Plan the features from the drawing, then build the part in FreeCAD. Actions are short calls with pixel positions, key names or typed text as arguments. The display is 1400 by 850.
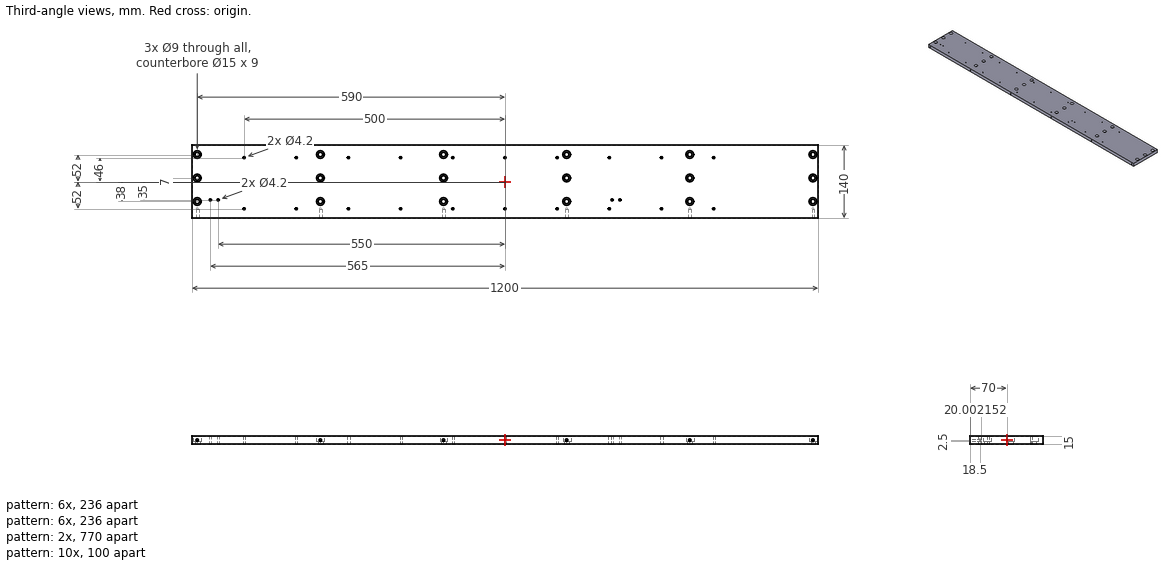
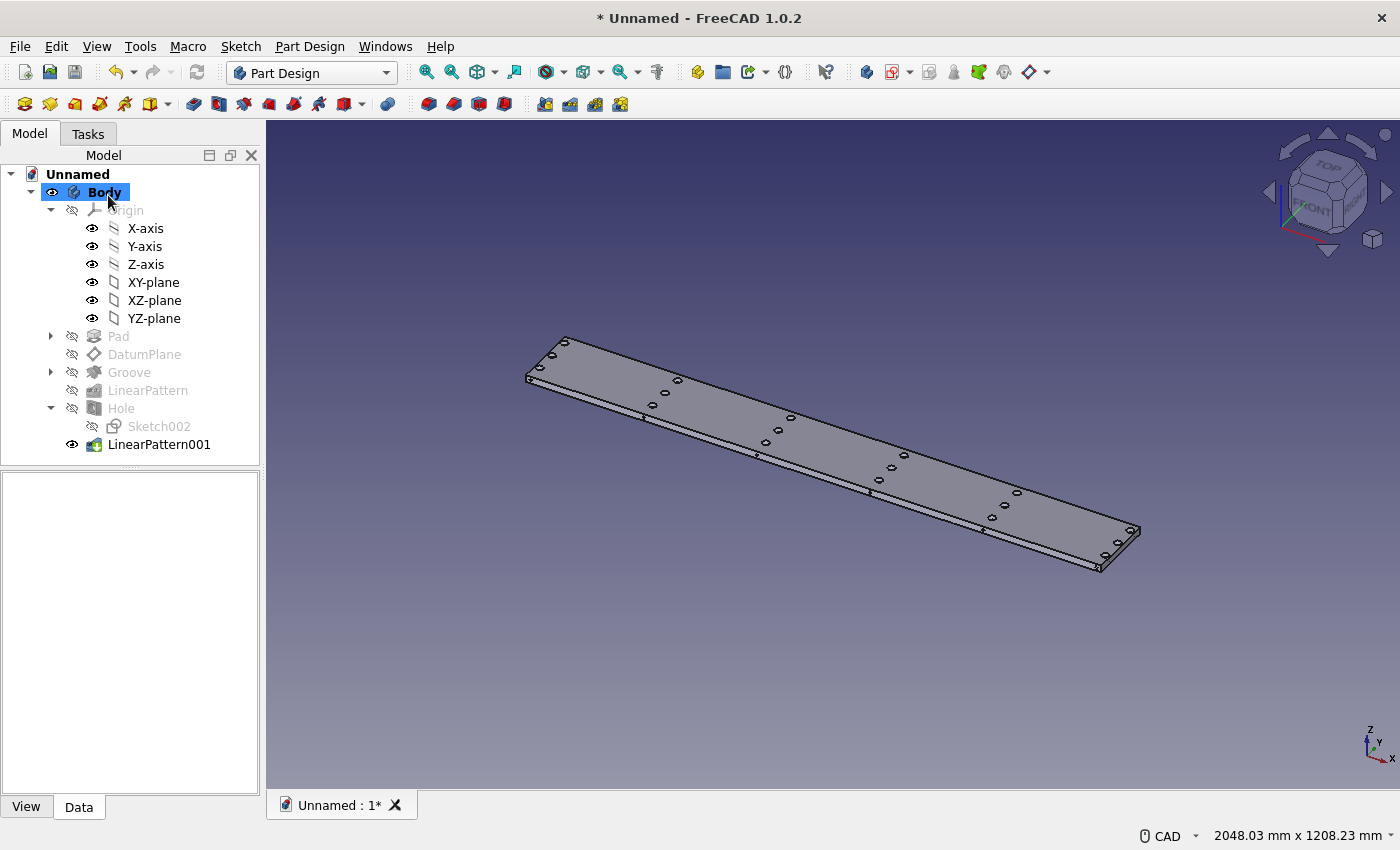
key(5)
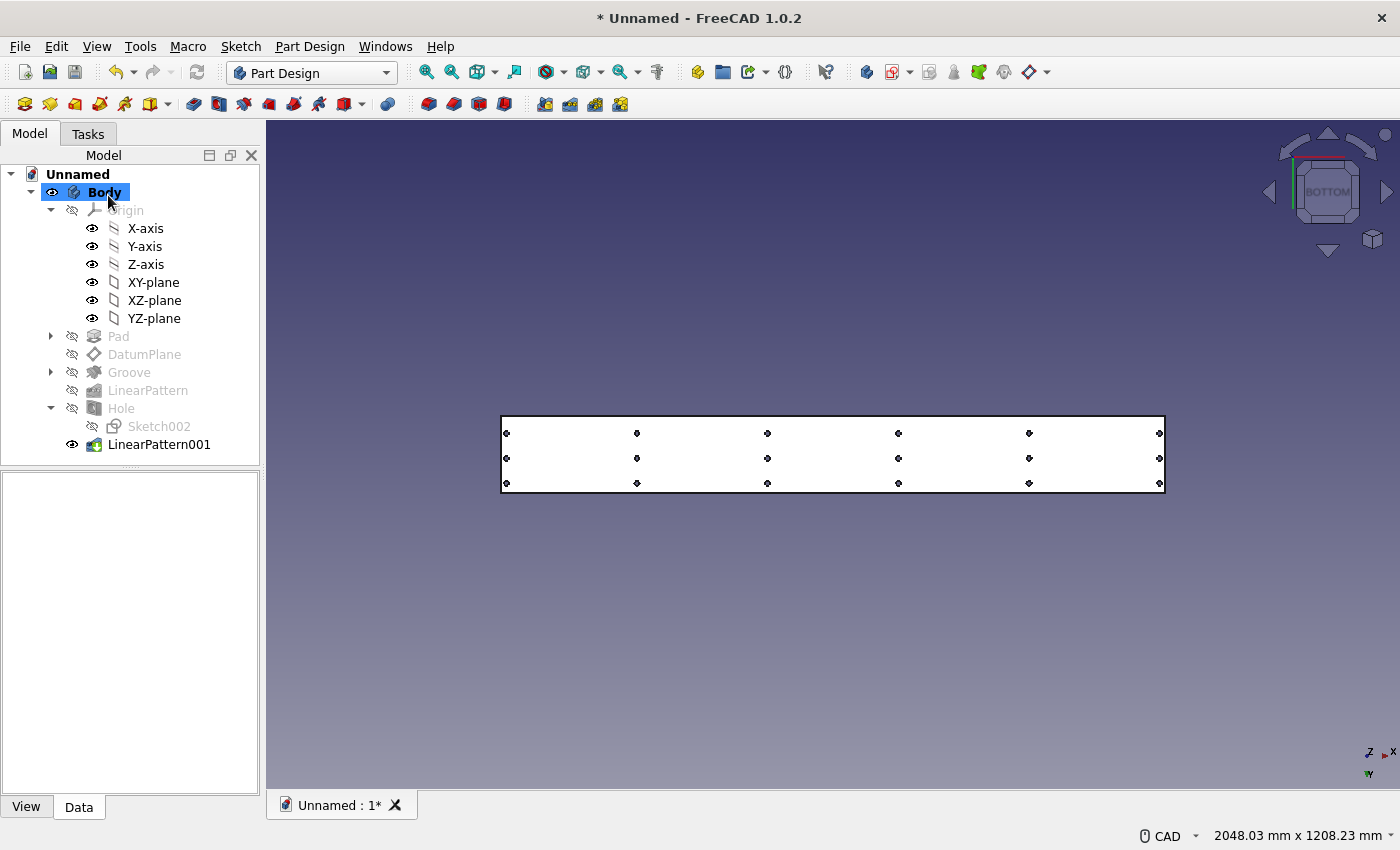
click(1118, 453)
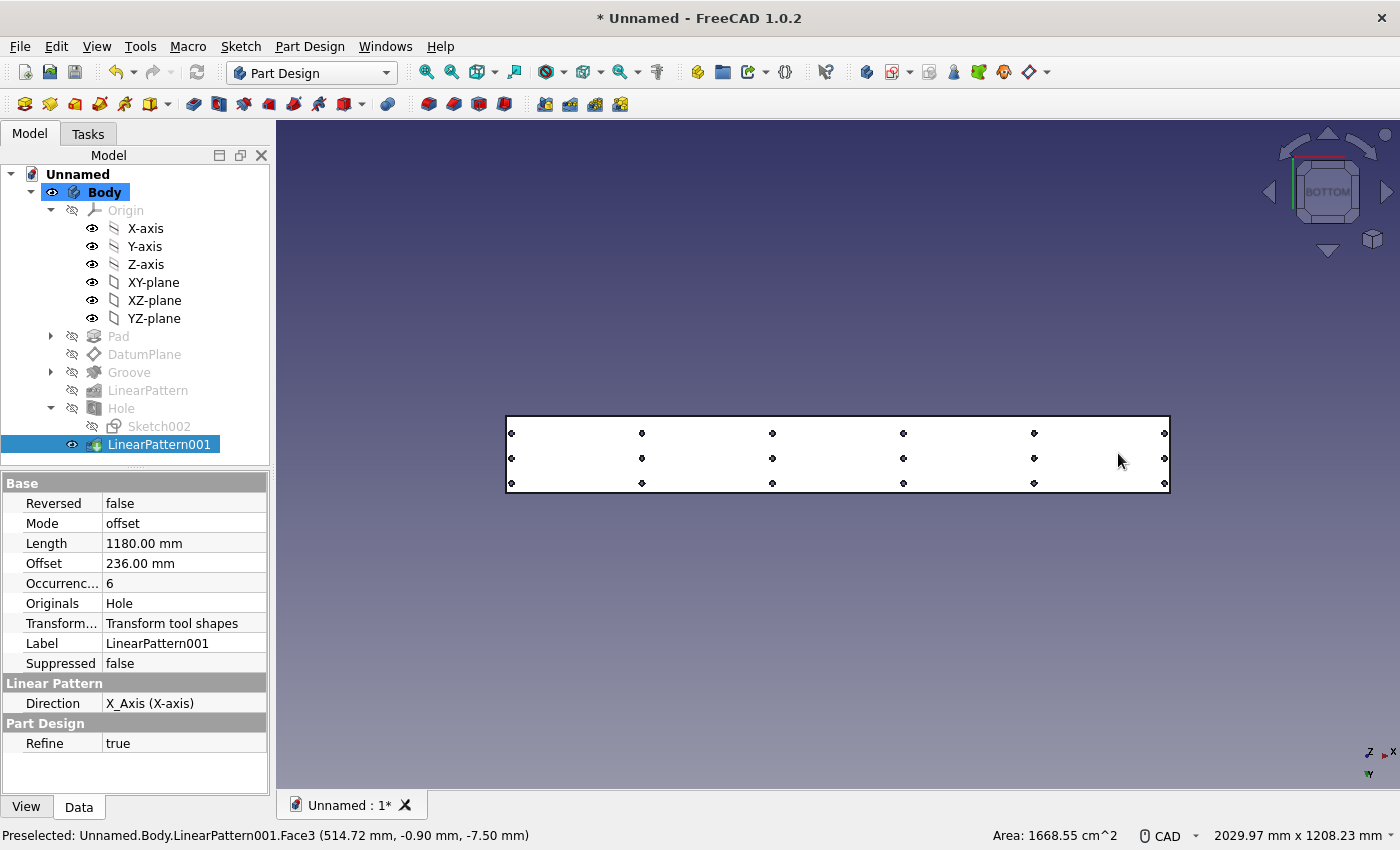
click(892, 72)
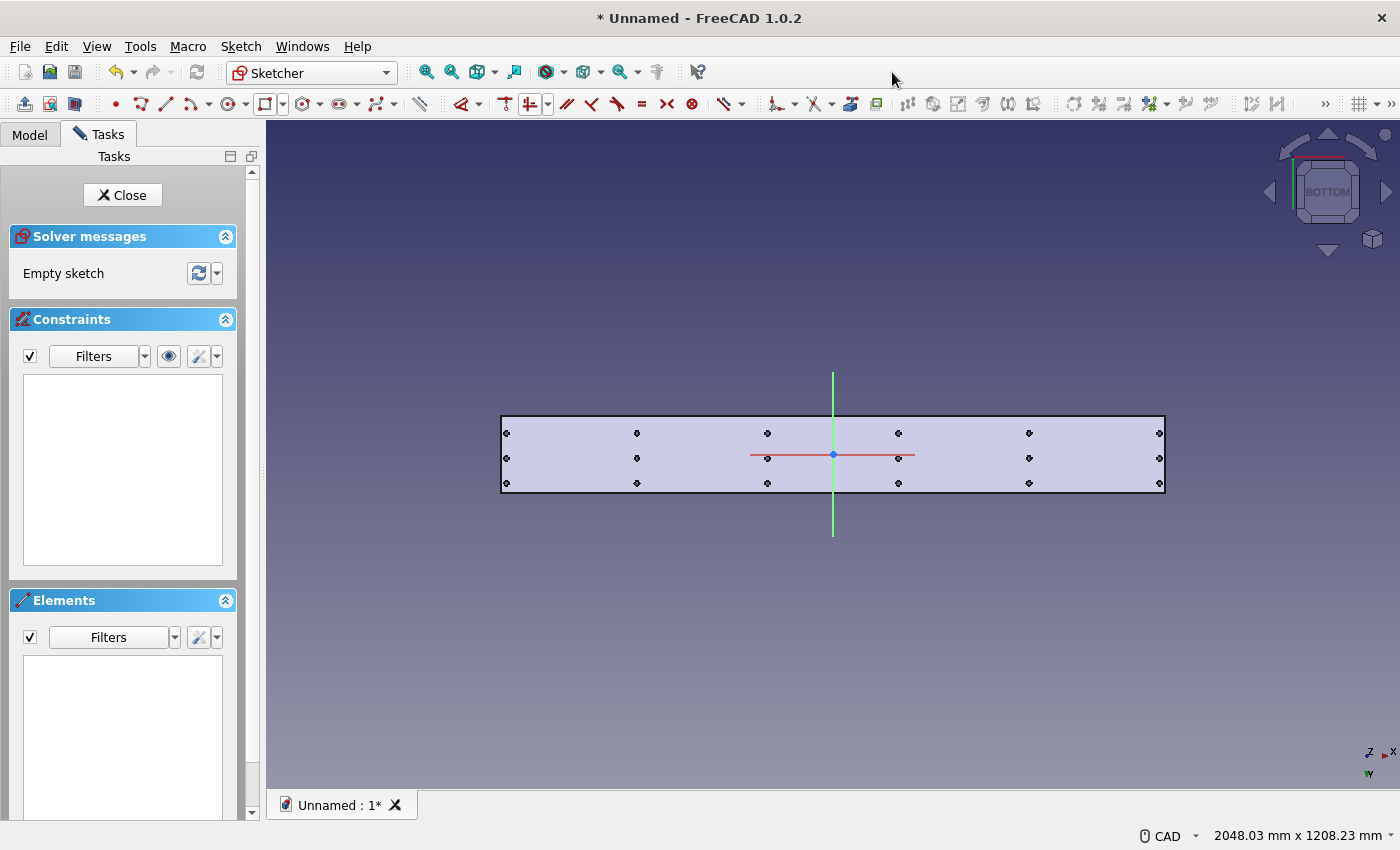
scroll(512, 434, up, 15)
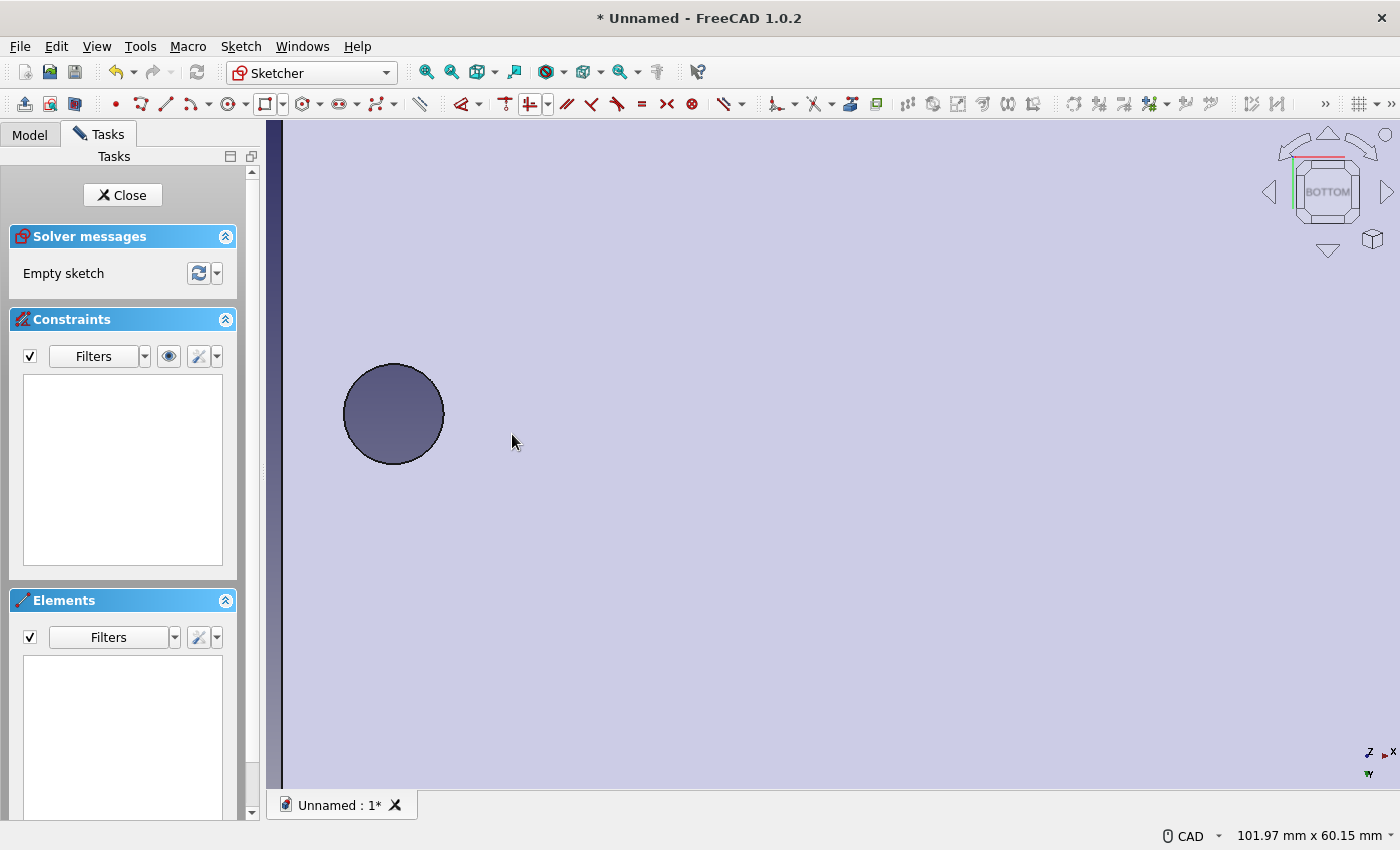
scroll(751, 445, up, 6)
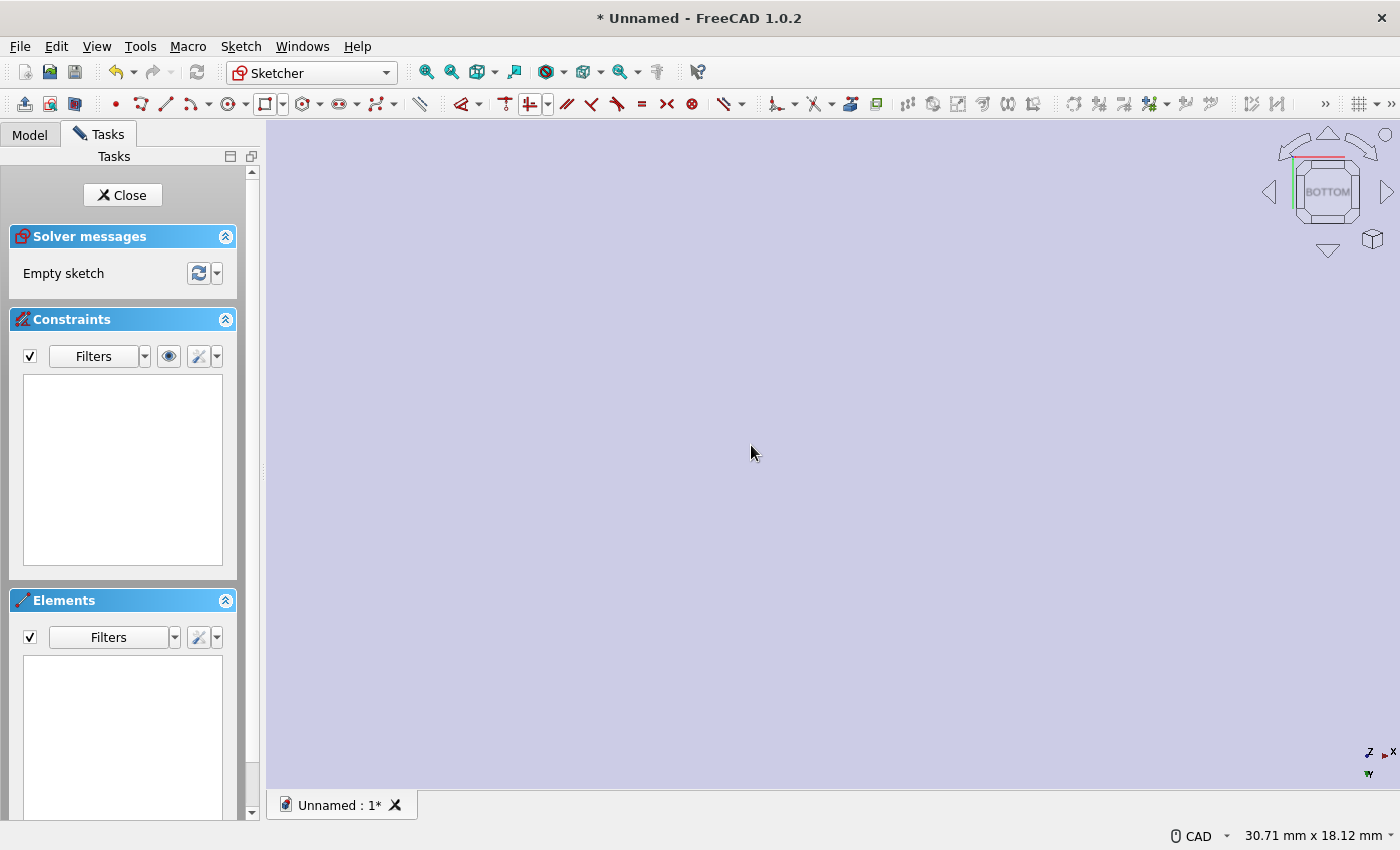
click(228, 104)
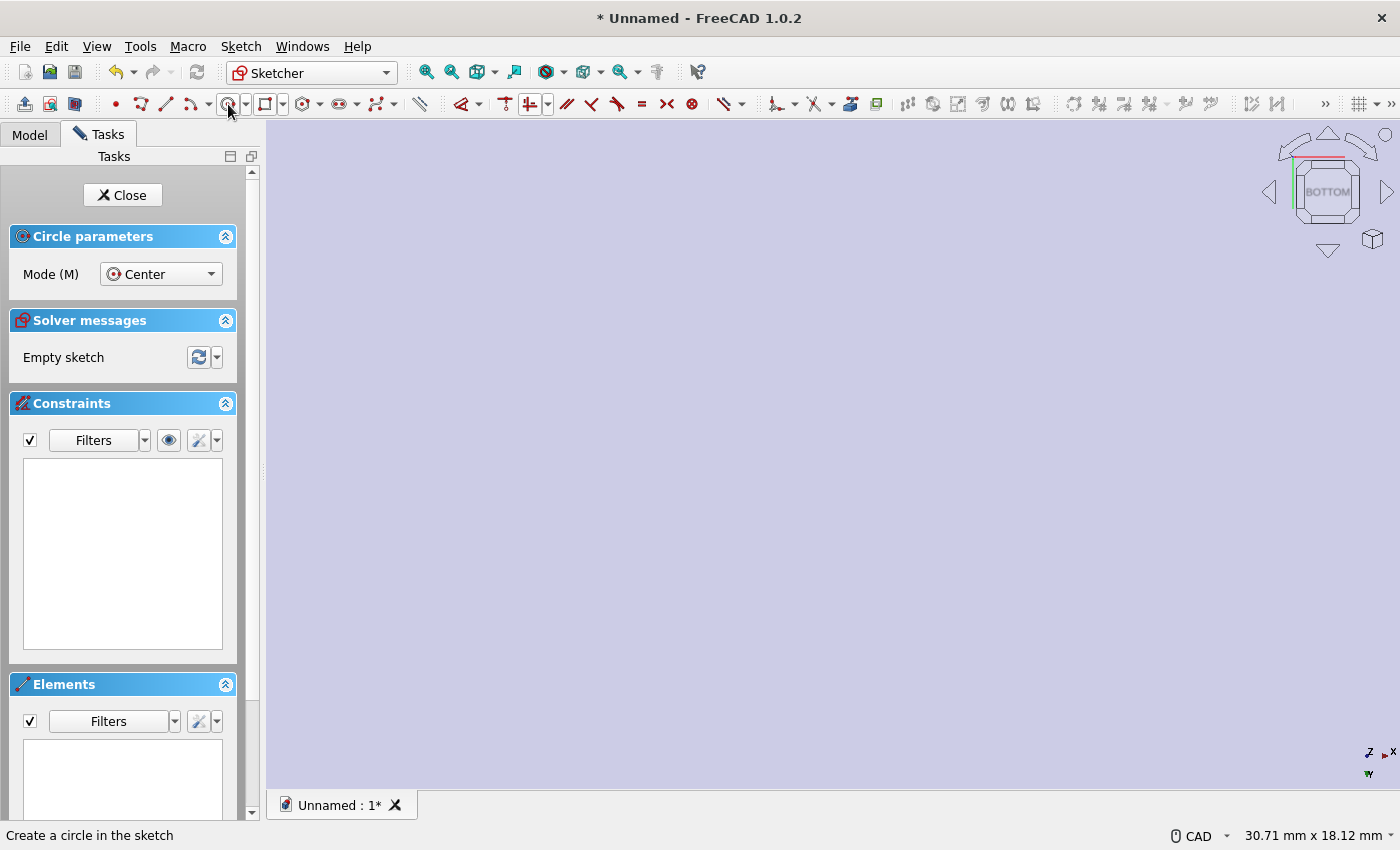
click(1041, 452)
move(1096, 397)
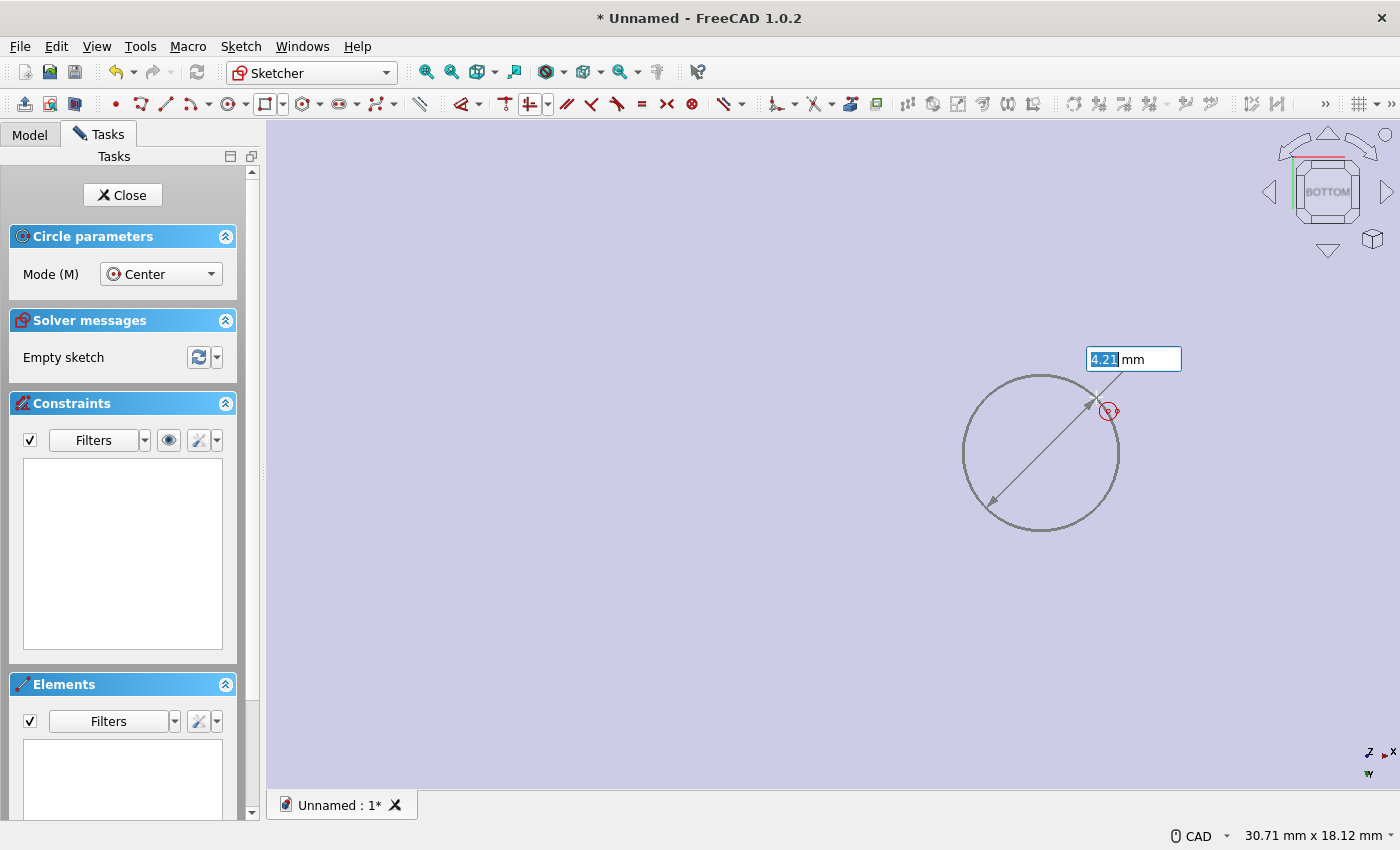
text(4.2)
key(Return)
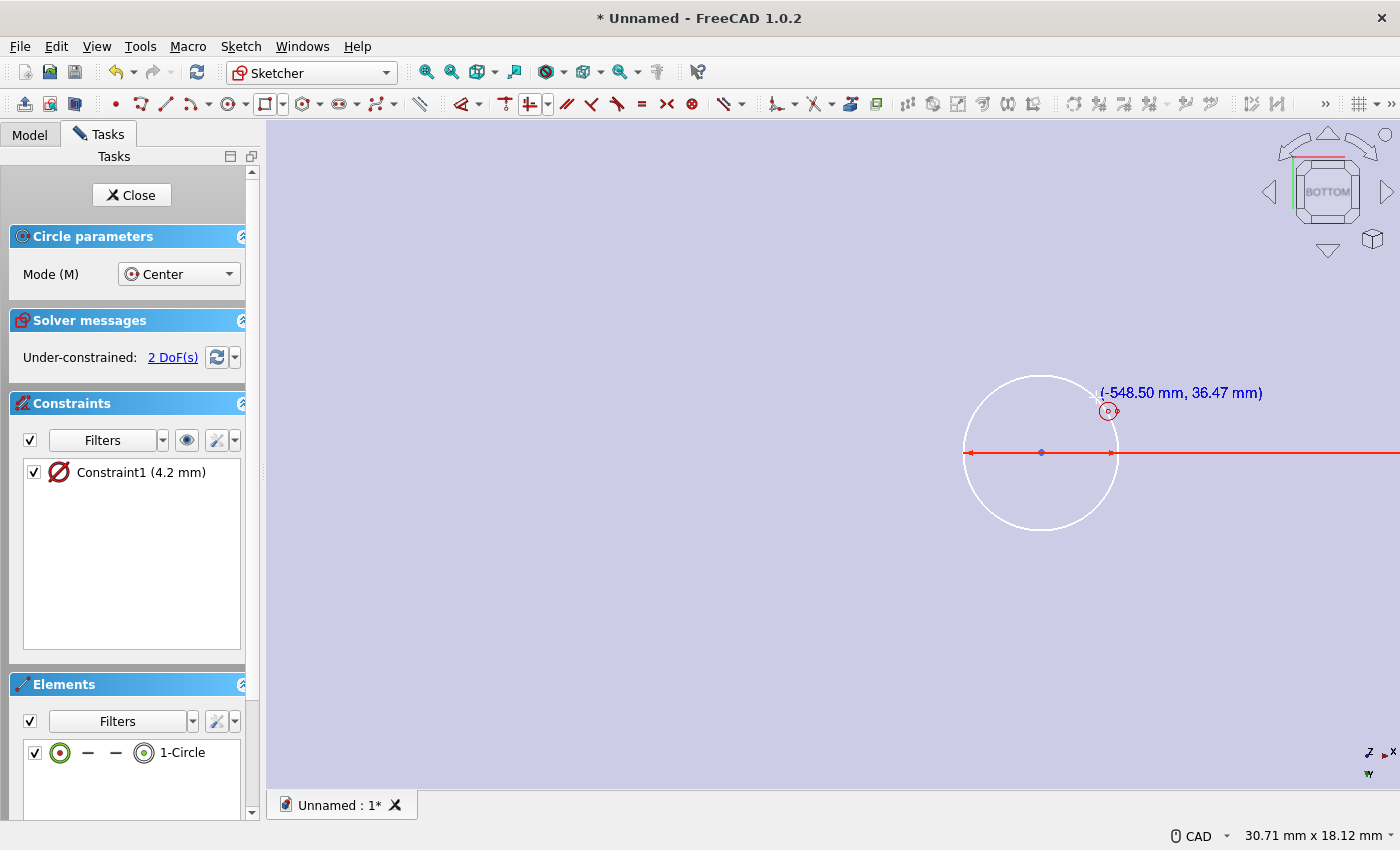
click(487, 452)
move(542, 397)